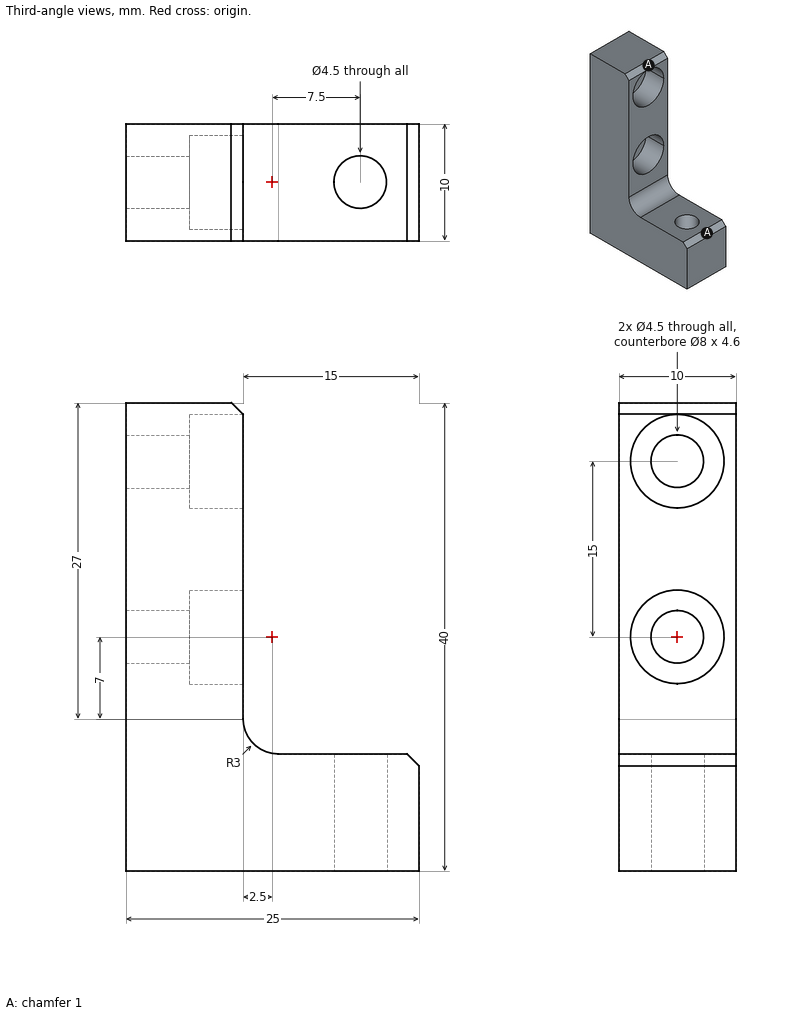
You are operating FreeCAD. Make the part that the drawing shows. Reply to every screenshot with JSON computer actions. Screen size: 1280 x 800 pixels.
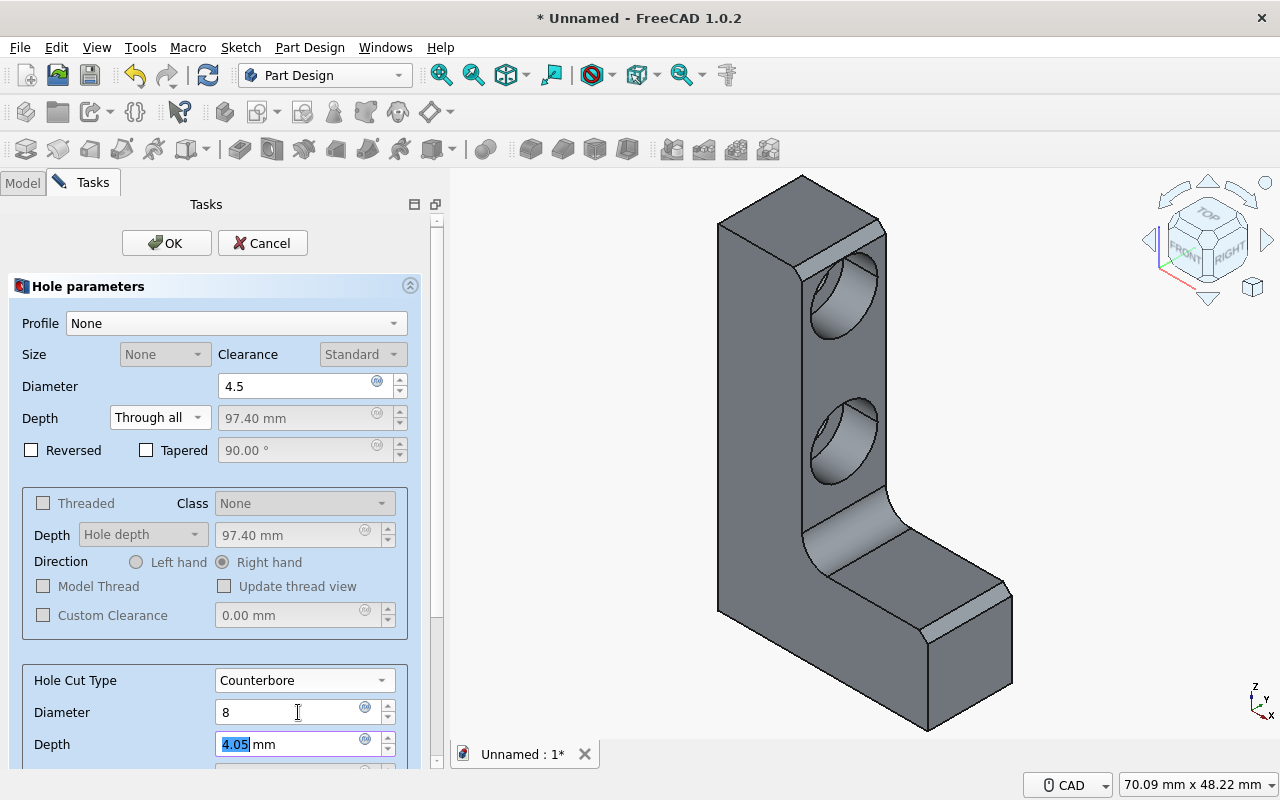
{"action": "type", "text": "4.6"}
{"action": "key", "text": "Tab"}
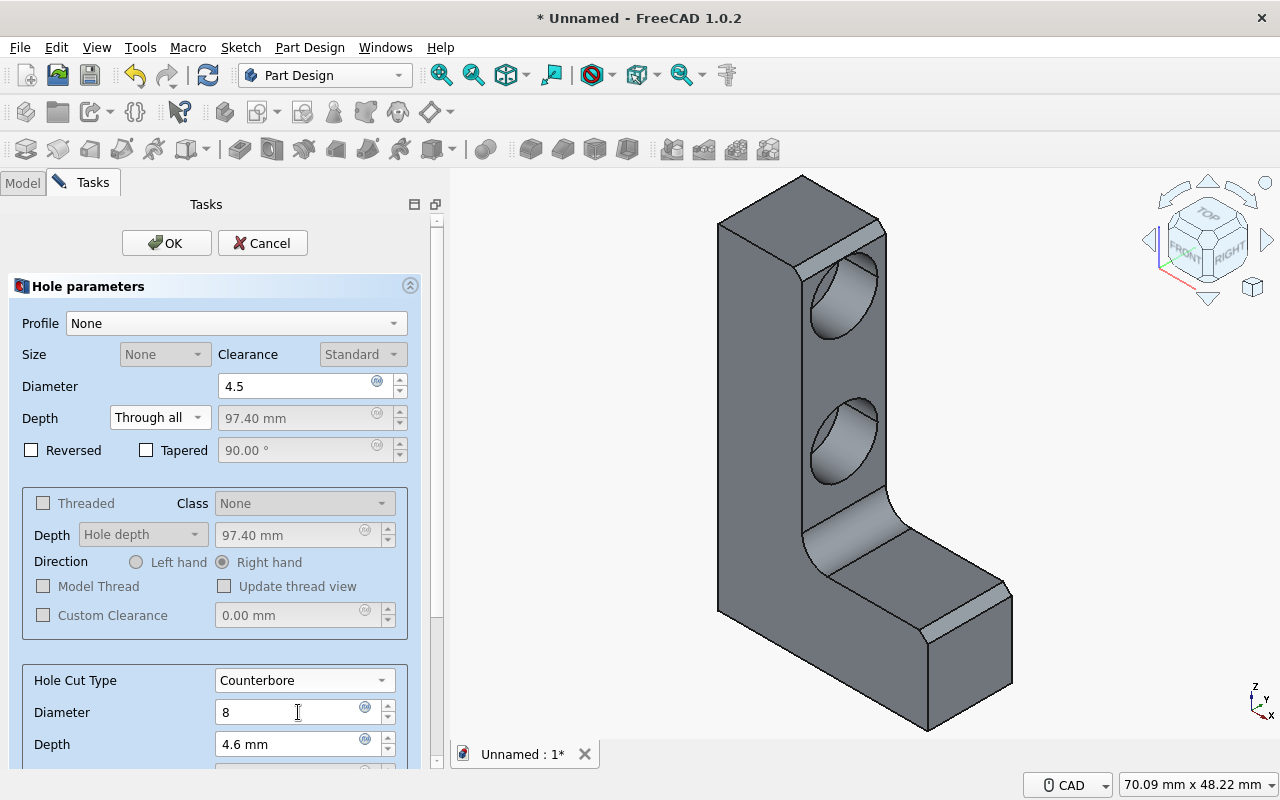
{"action": "left_click", "coordinate": [167, 243]}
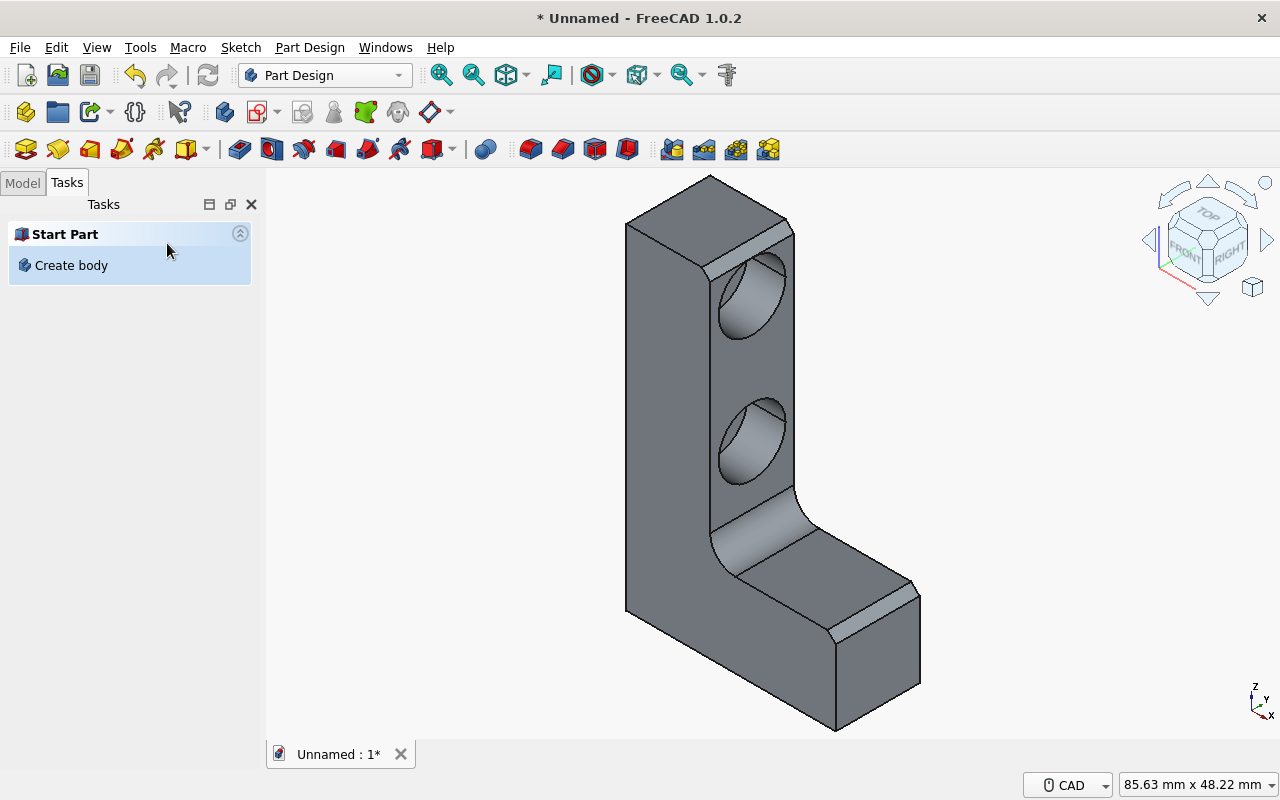
{"action": "left_click", "coordinate": [823, 578]}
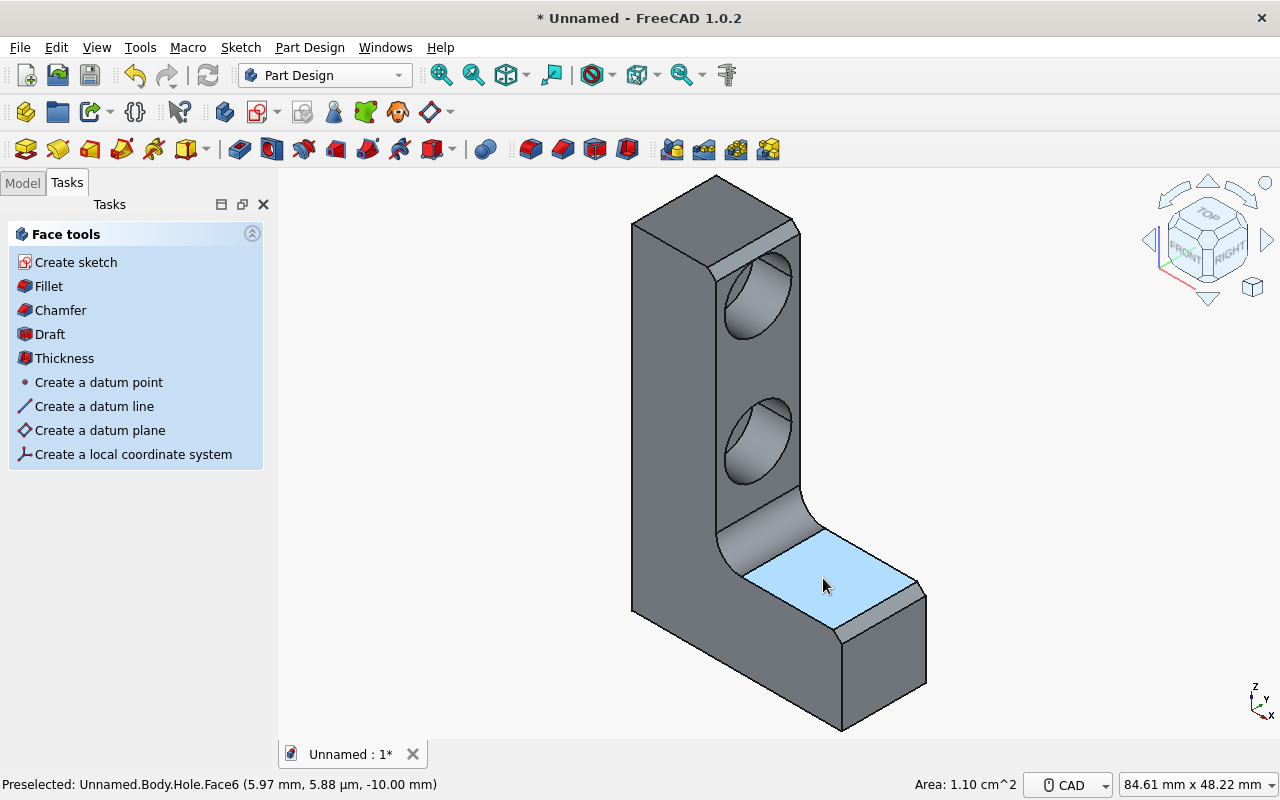
{"action": "left_click", "coordinate": [258, 112]}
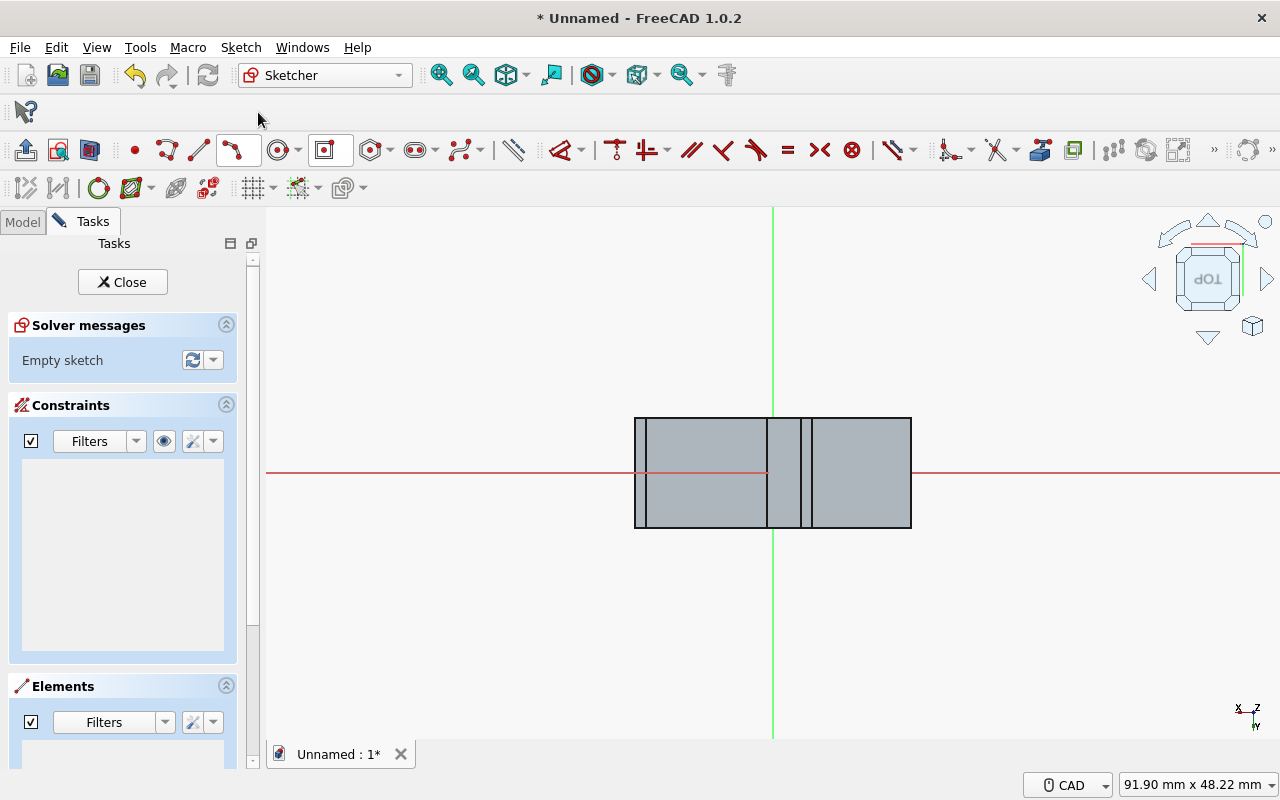
{"action": "scroll", "coordinate": [723, 473], "scroll_direction": "up", "scroll_amount": 8}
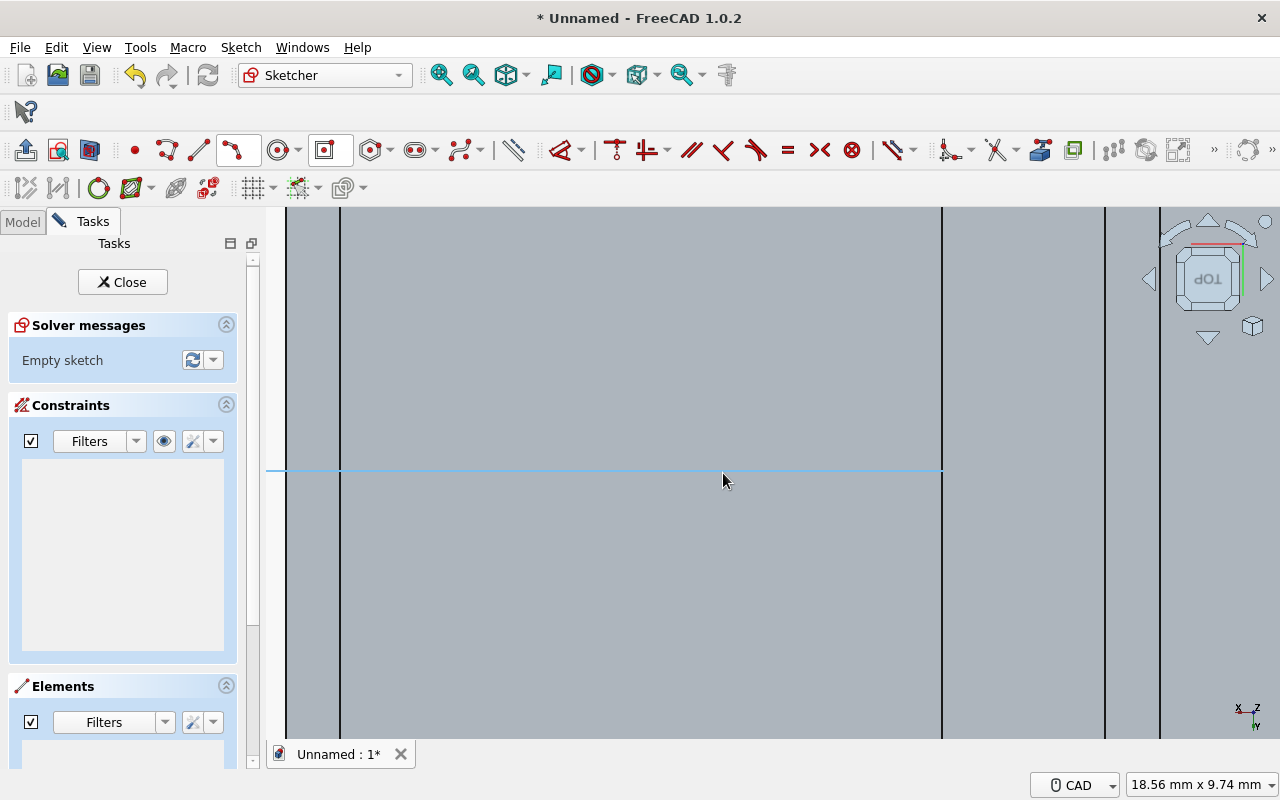
{"action": "key", "text": "g c"}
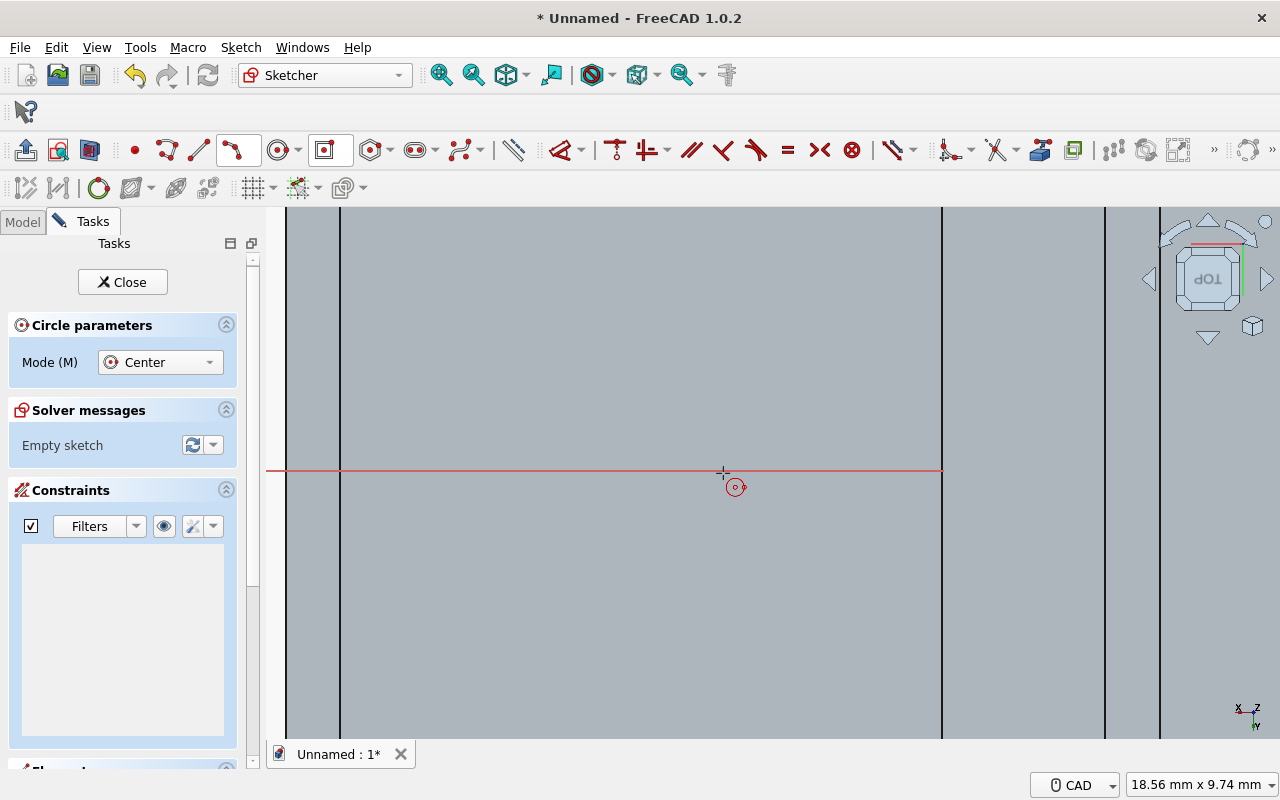
{"action": "left_click", "coordinate": [559, 471]}
{"action": "mouse_move", "coordinate": [646, 384]}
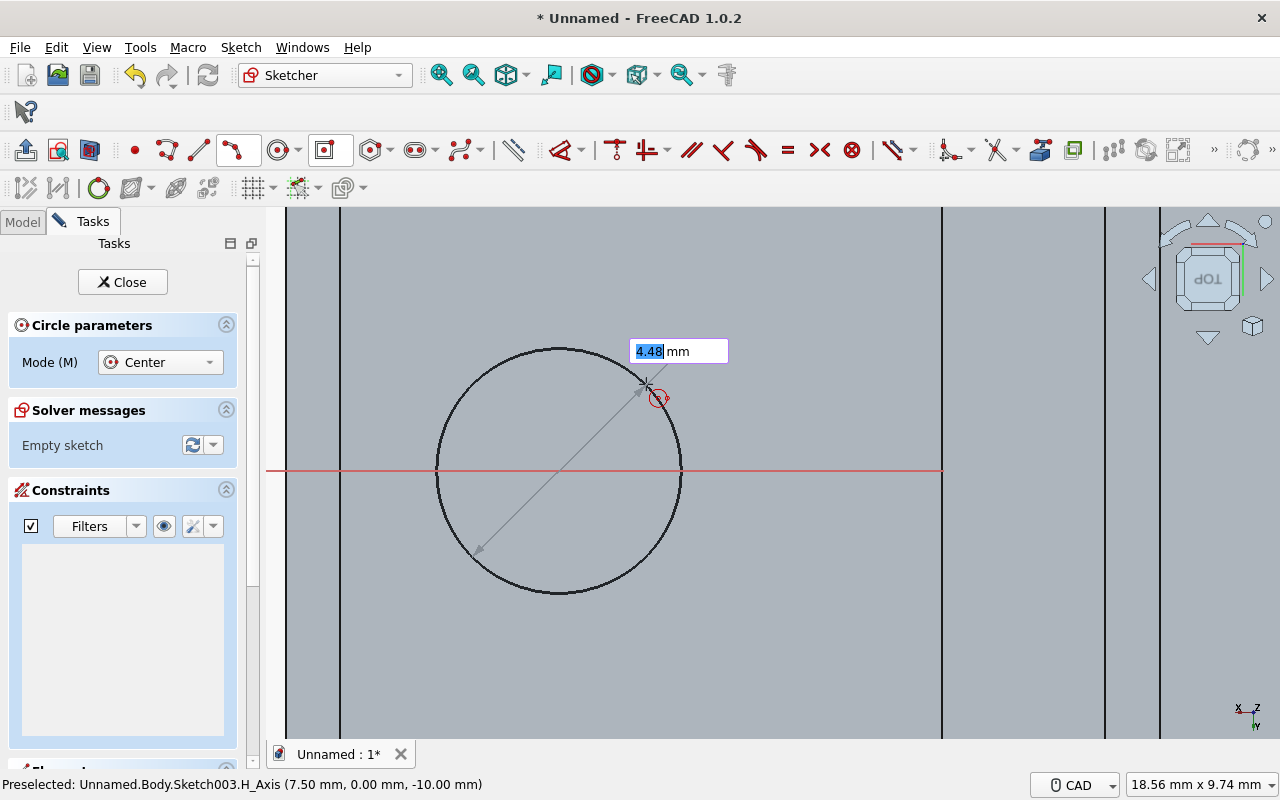
{"action": "type", "text": "4.5"}
{"action": "key", "text": "Return"}
{"action": "key", "text": "Escape"}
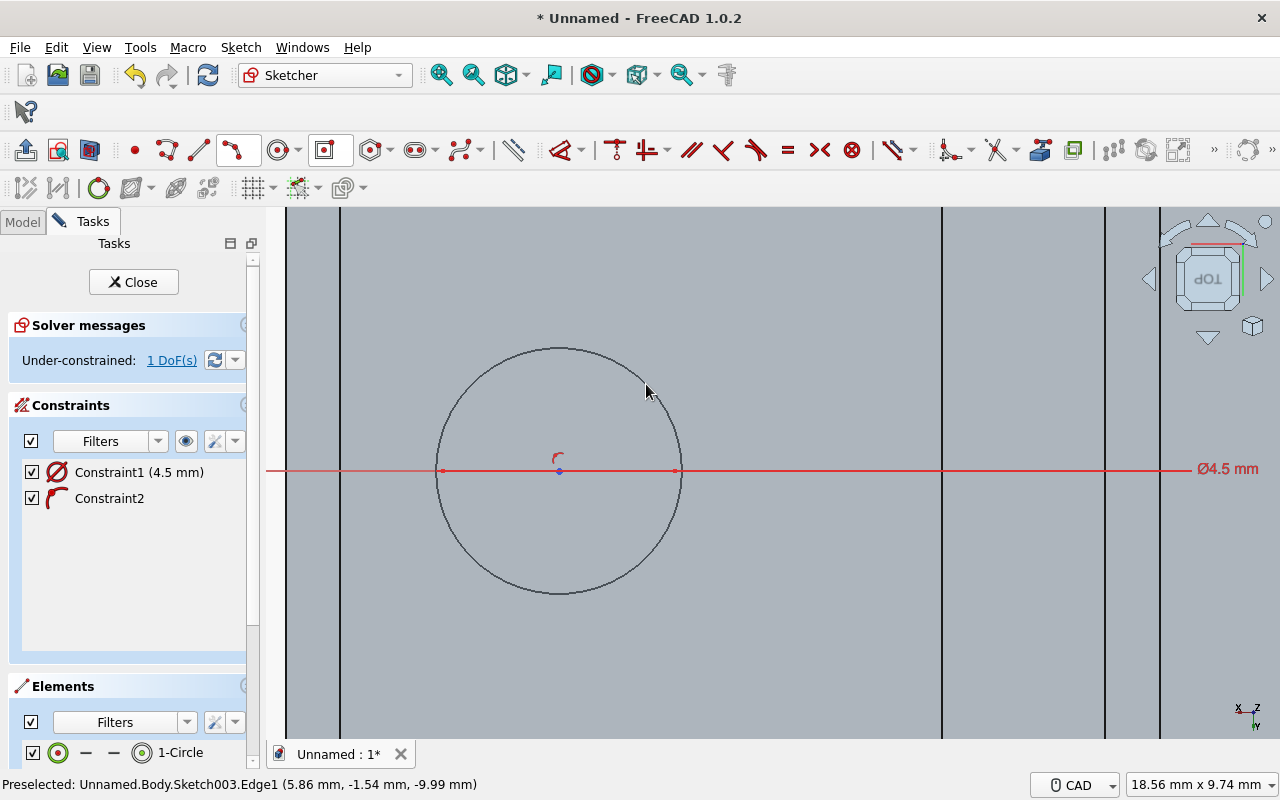
{"action": "left_click", "coordinate": [560, 150]}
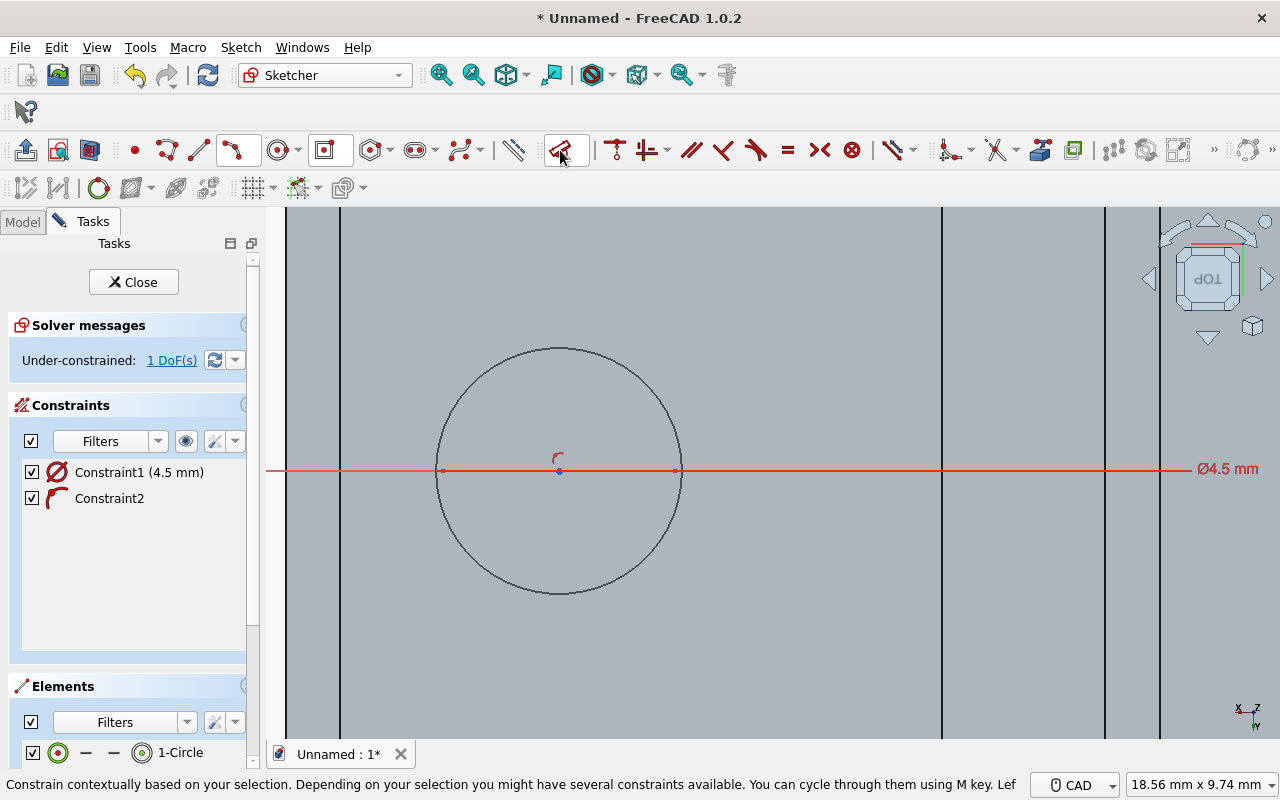
{"action": "left_click", "coordinate": [559, 471]}
{"action": "left_click", "coordinate": [764, 505]}